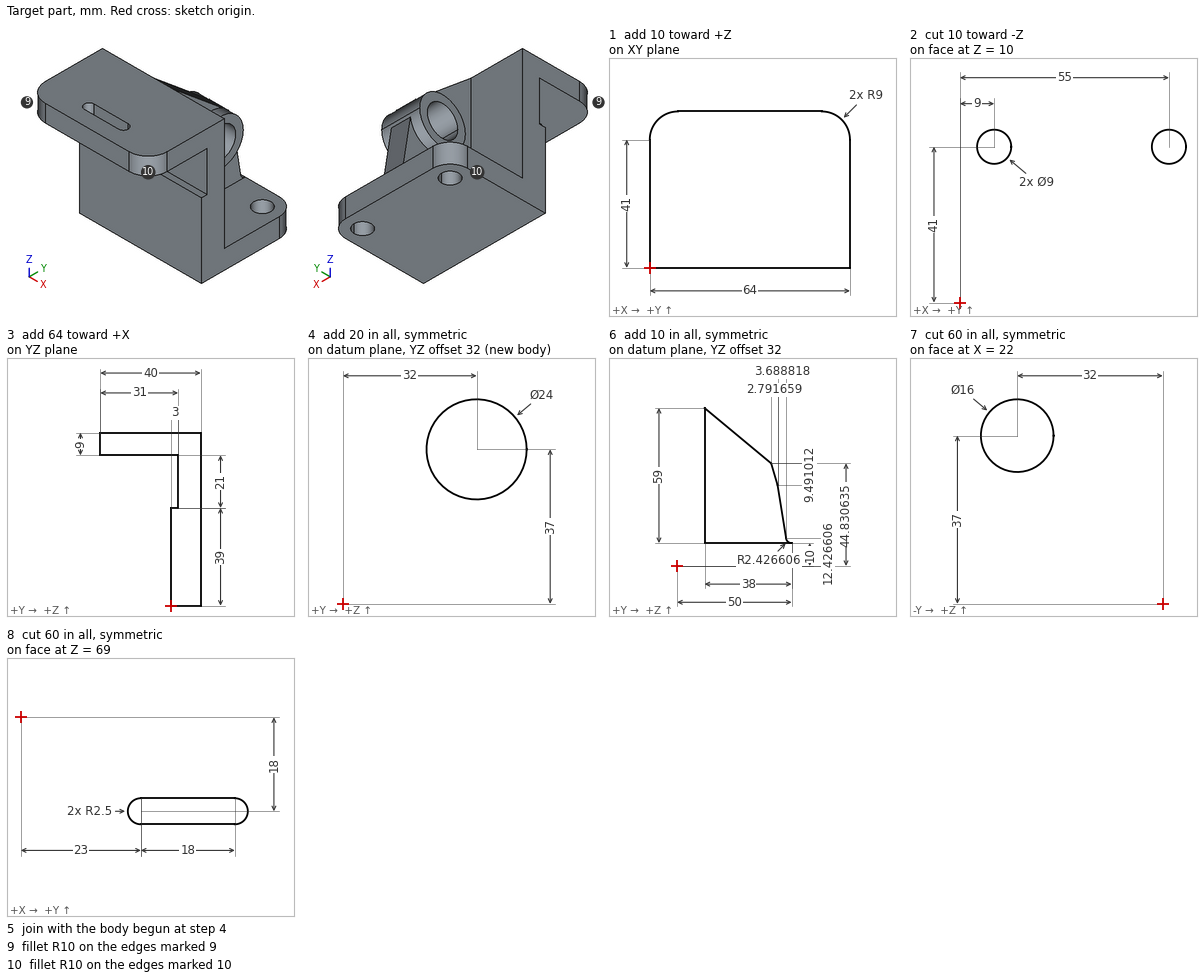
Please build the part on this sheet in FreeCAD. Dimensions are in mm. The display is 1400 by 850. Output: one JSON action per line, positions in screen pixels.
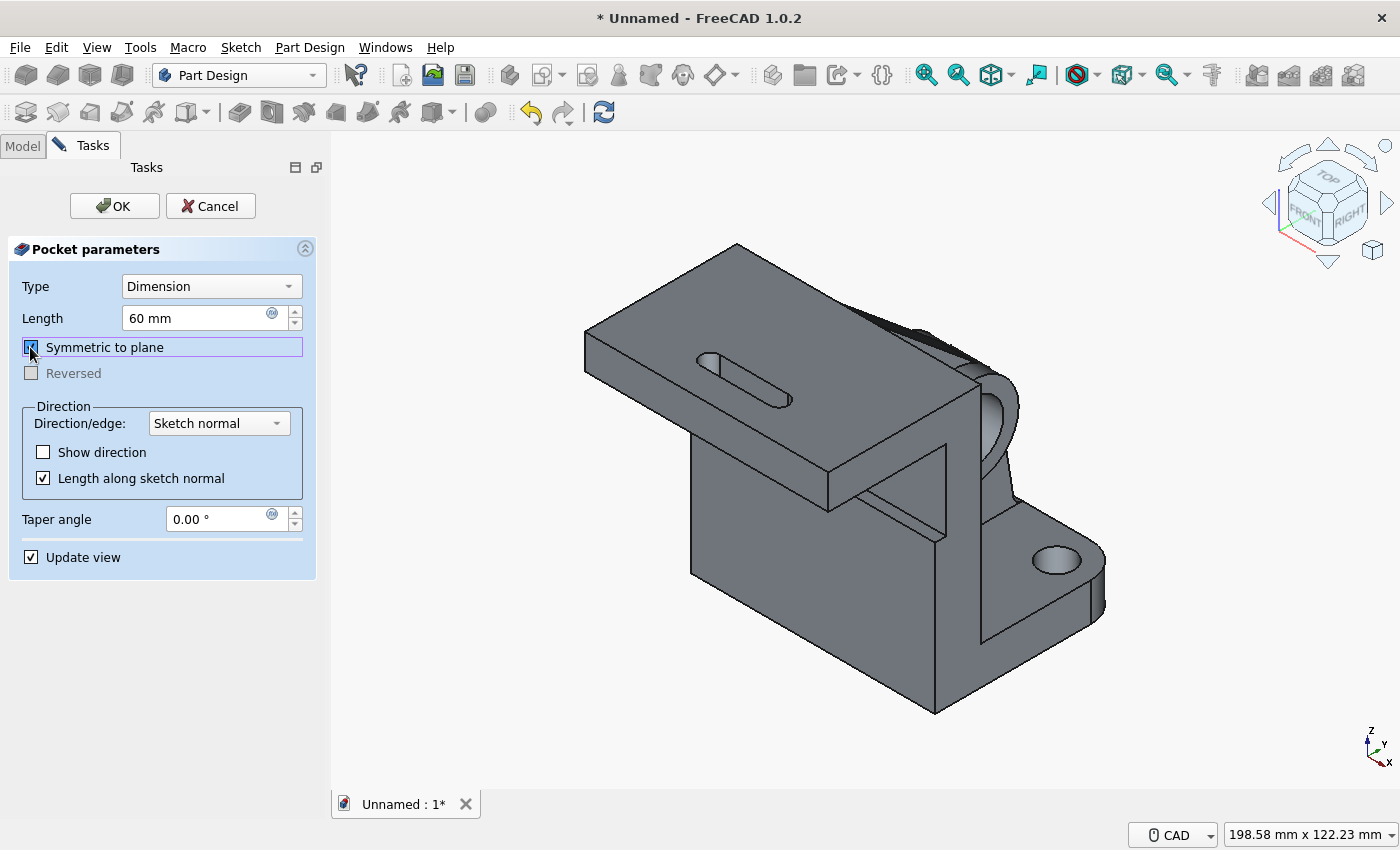
{"action": "left_click", "coordinate": [115, 206]}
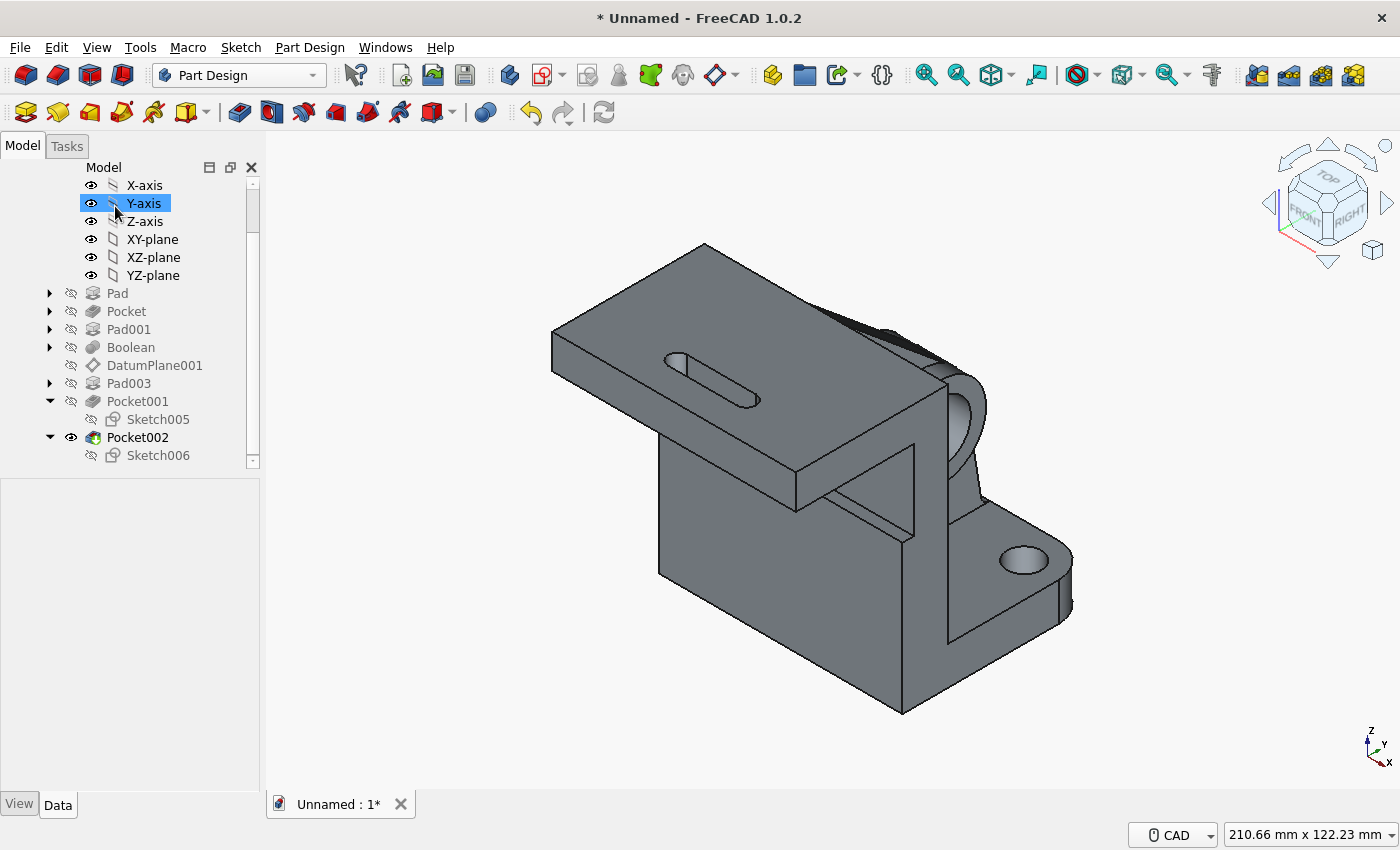
{"action": "key", "text": "2"}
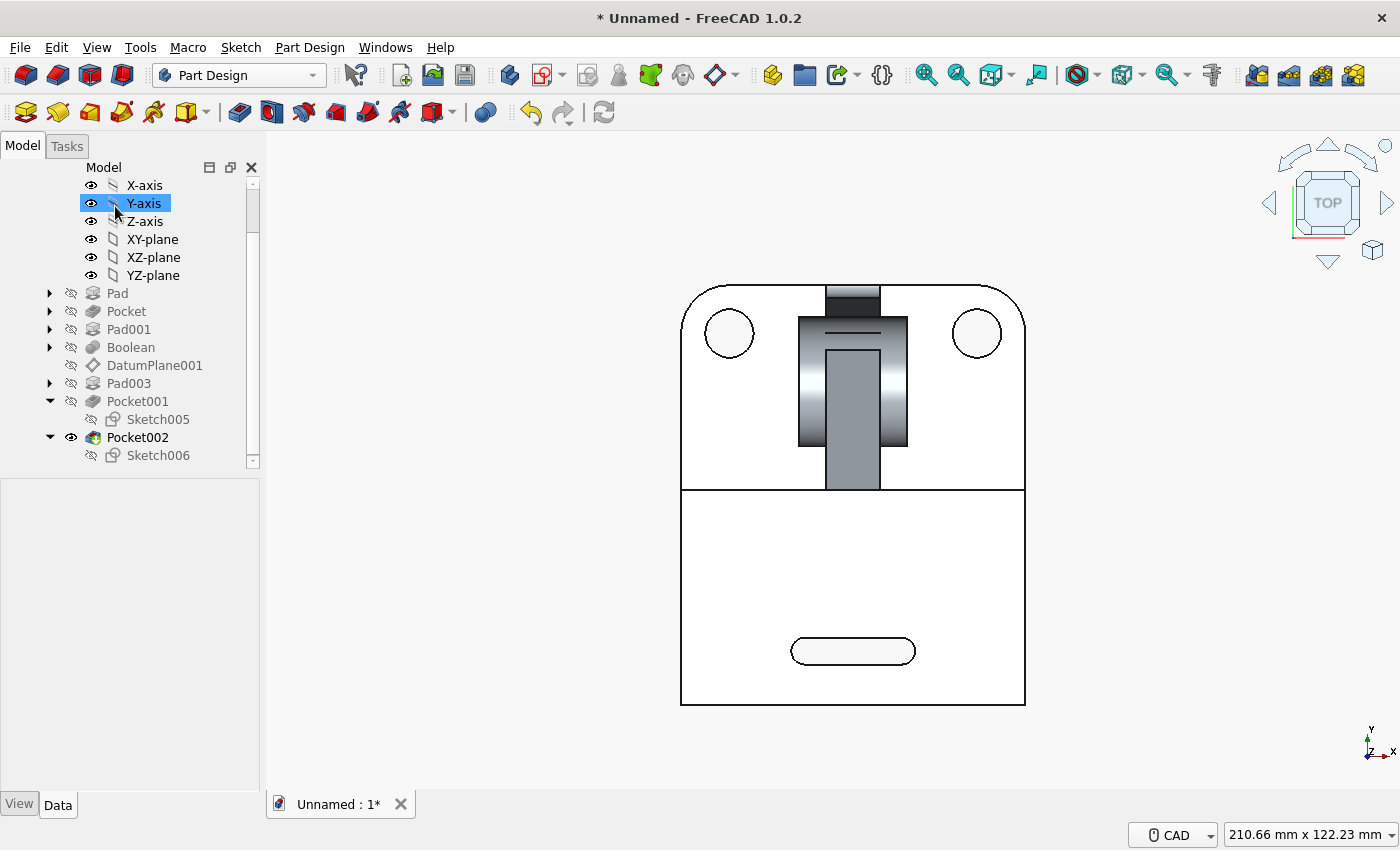
{"action": "key", "text": "0"}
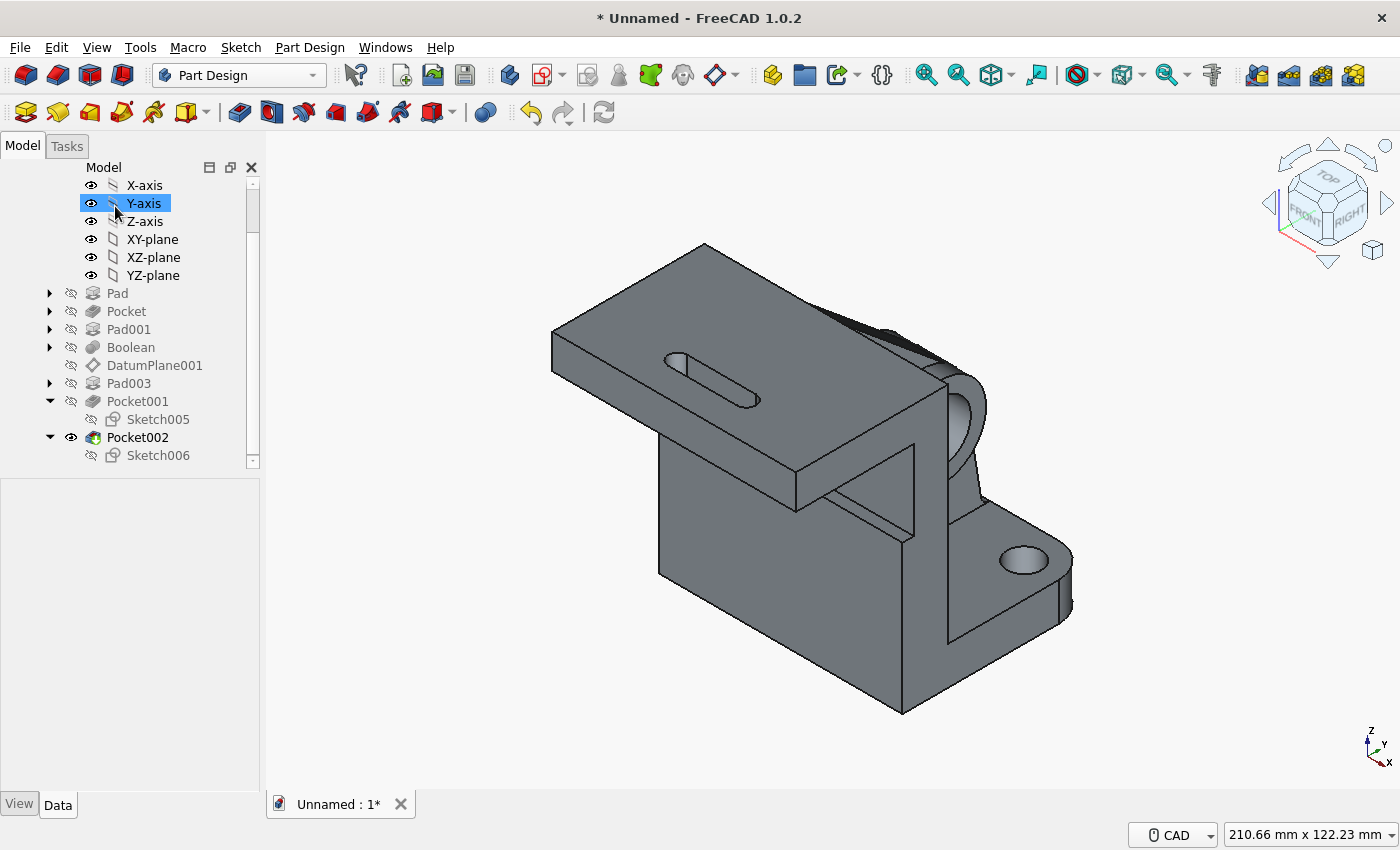
{"action": "key", "text": "1"}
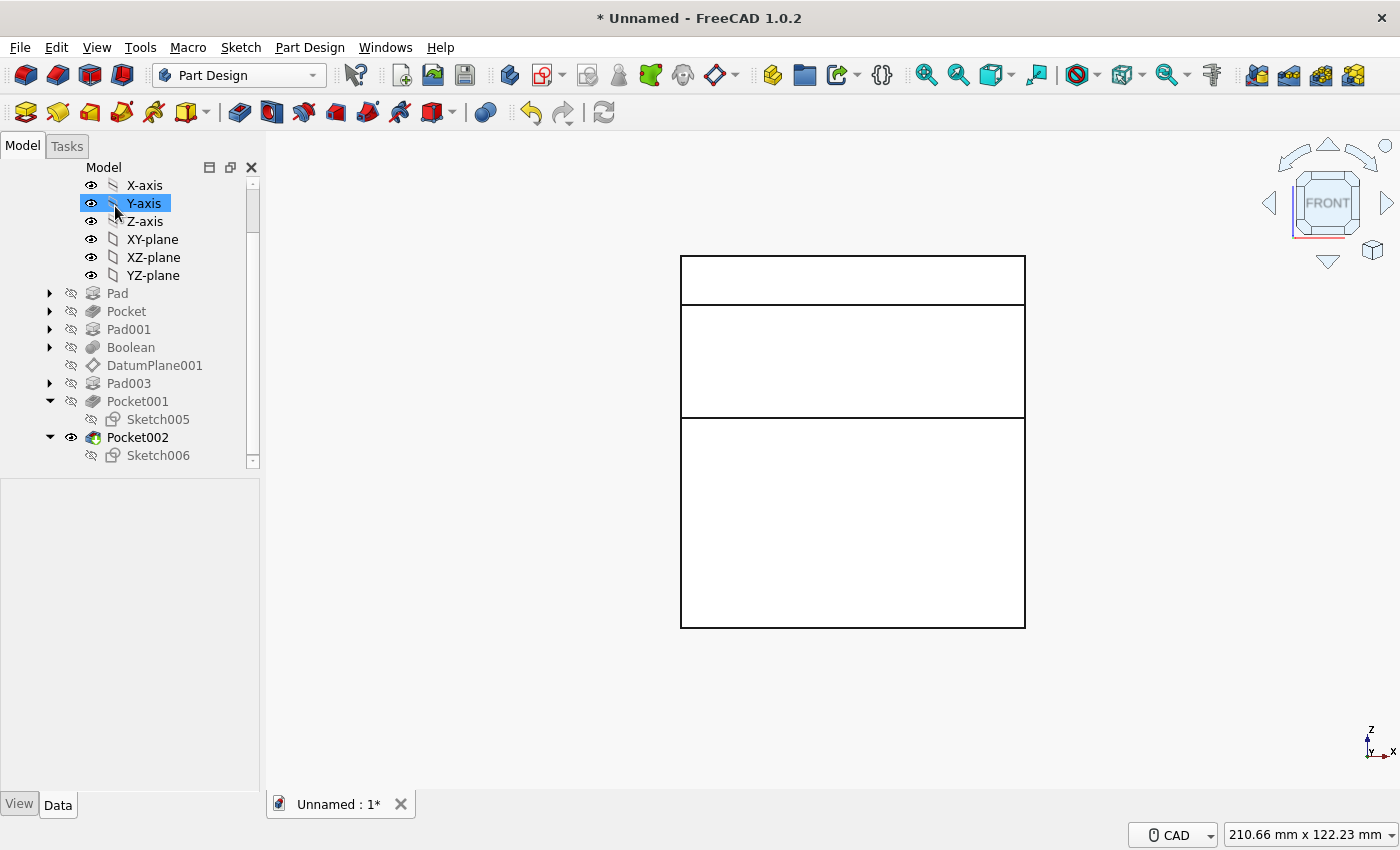
{"action": "left_click", "coordinate": [681, 280]}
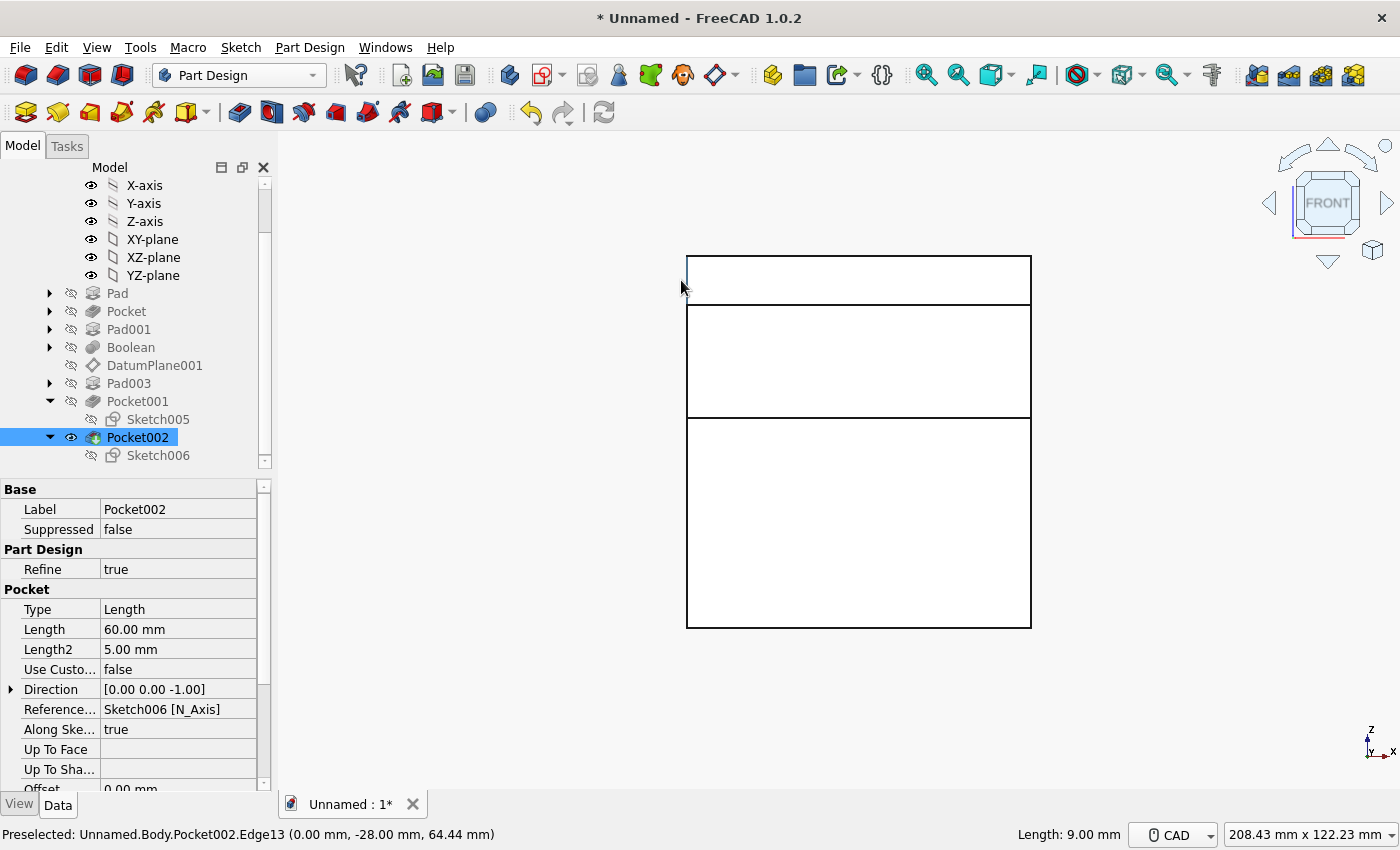
{"action": "left_click", "coordinate": [26, 76]}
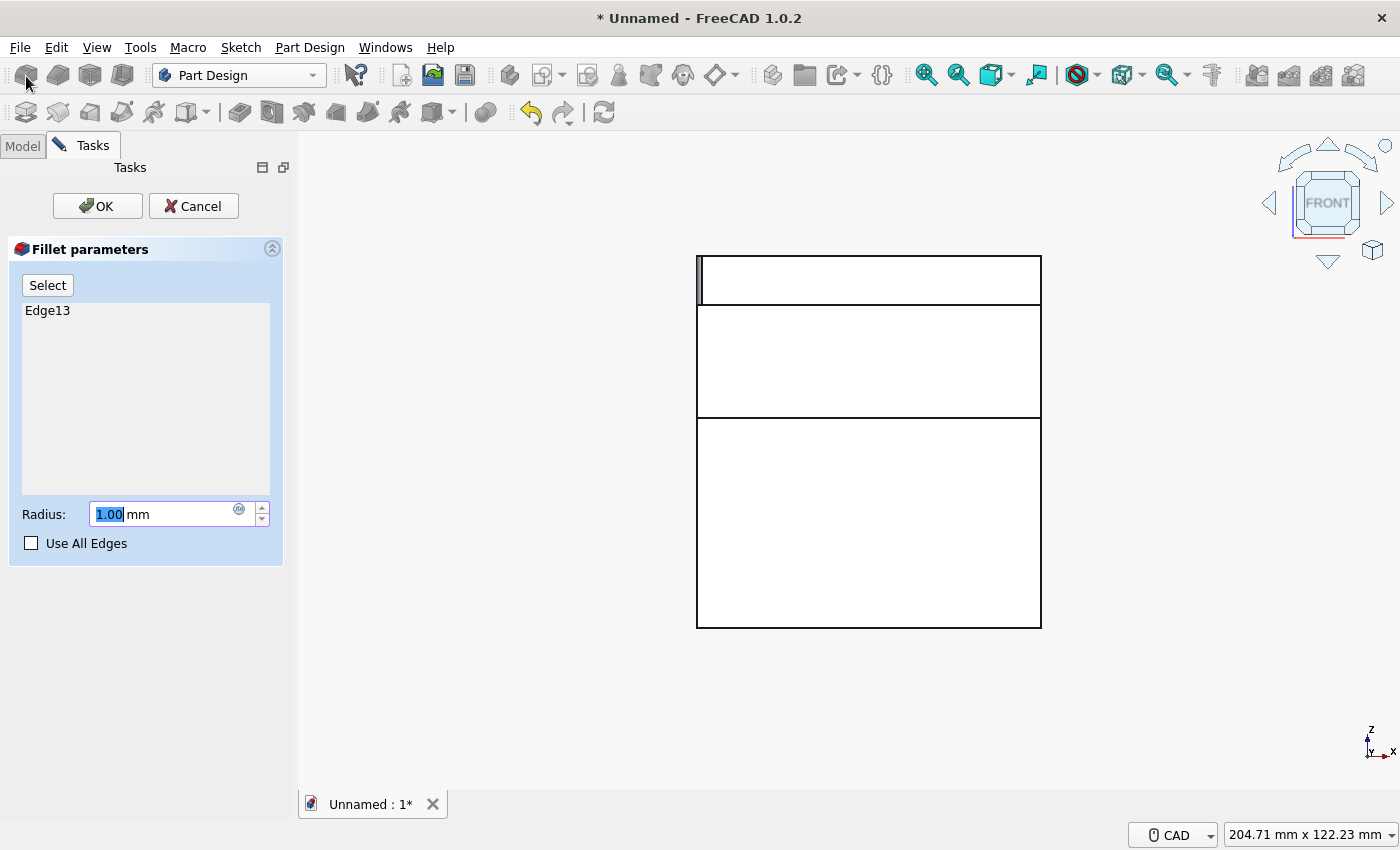
{"action": "type", "text": "10"}
{"action": "key", "text": "Tab"}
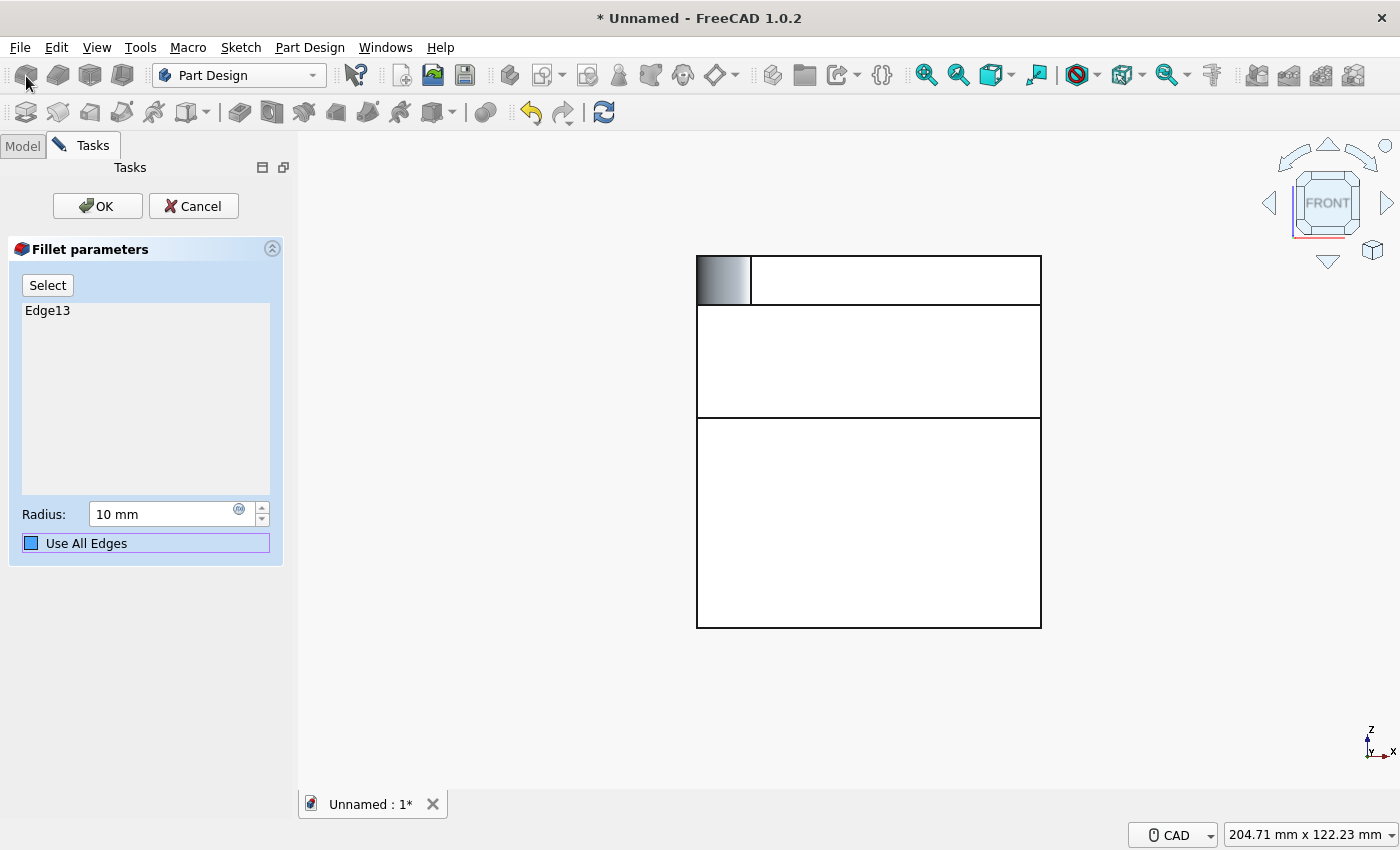
{"action": "left_click", "coordinate": [98, 206]}